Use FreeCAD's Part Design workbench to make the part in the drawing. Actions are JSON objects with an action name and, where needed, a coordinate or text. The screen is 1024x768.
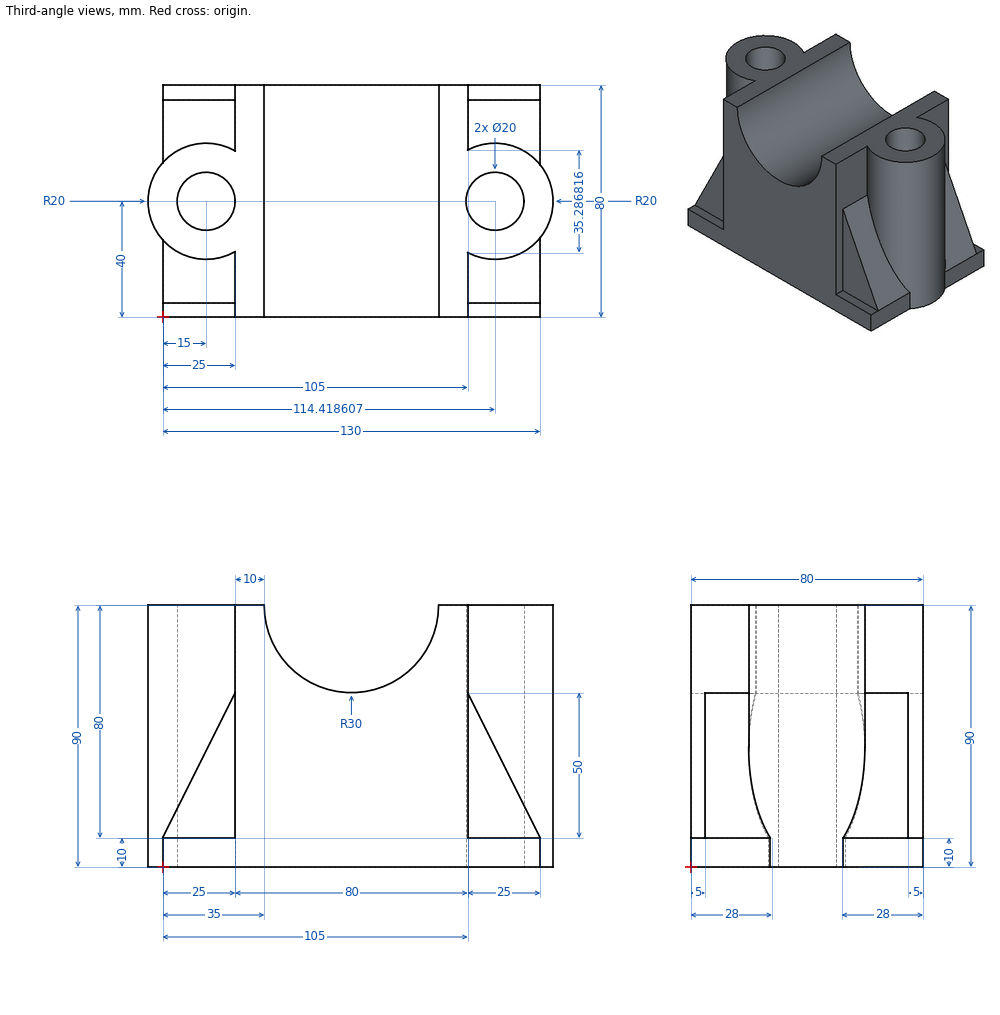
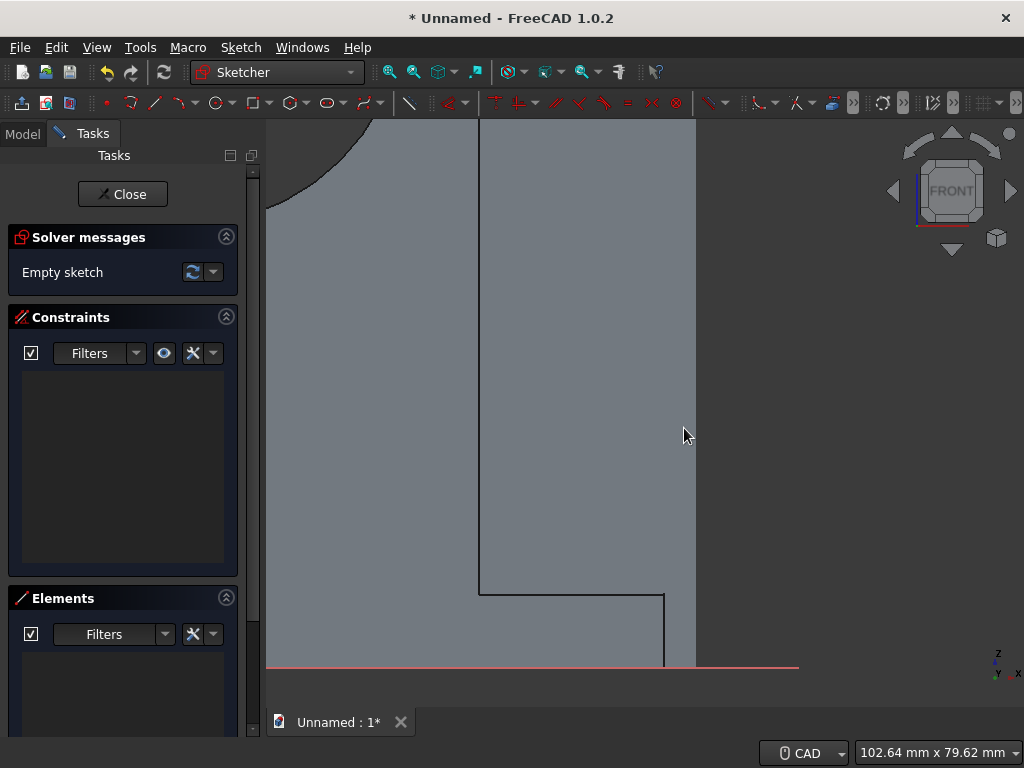
{"action": "left_click", "coordinate": [132, 104]}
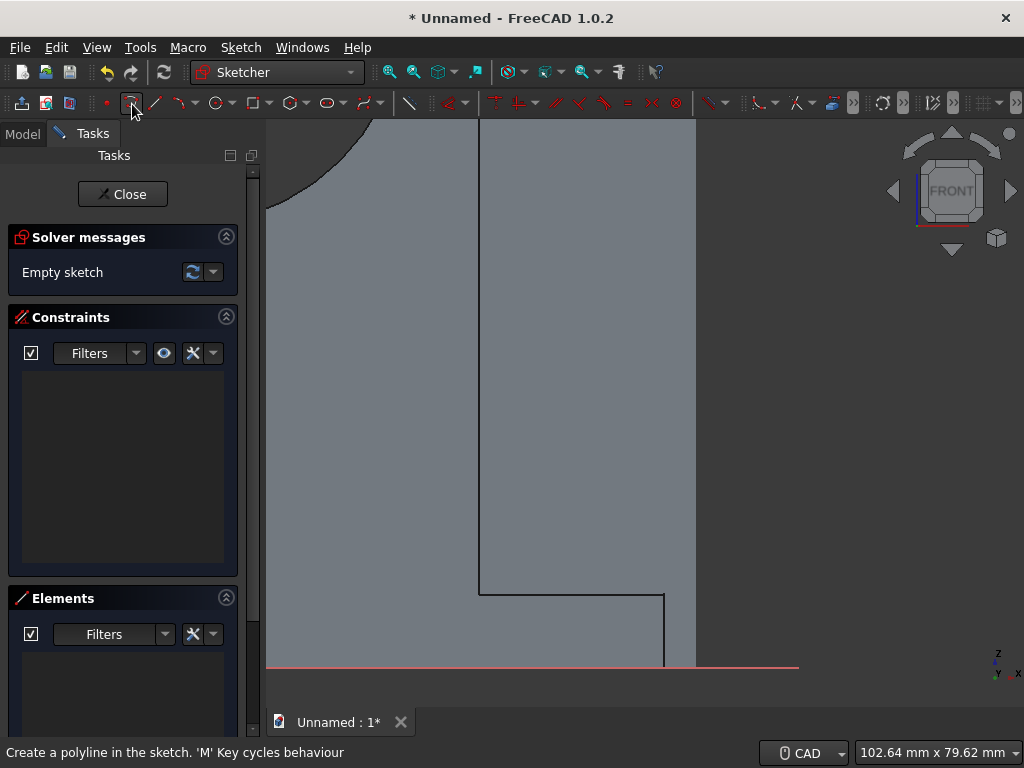
{"action": "left_click", "coordinate": [479, 594]}
{"action": "left_click", "coordinate": [664, 594]}
{"action": "left_click", "coordinate": [479, 225]}
{"action": "left_click", "coordinate": [479, 595]}
{"action": "key", "text": "Escape"}
{"action": "key", "text": "Escape"}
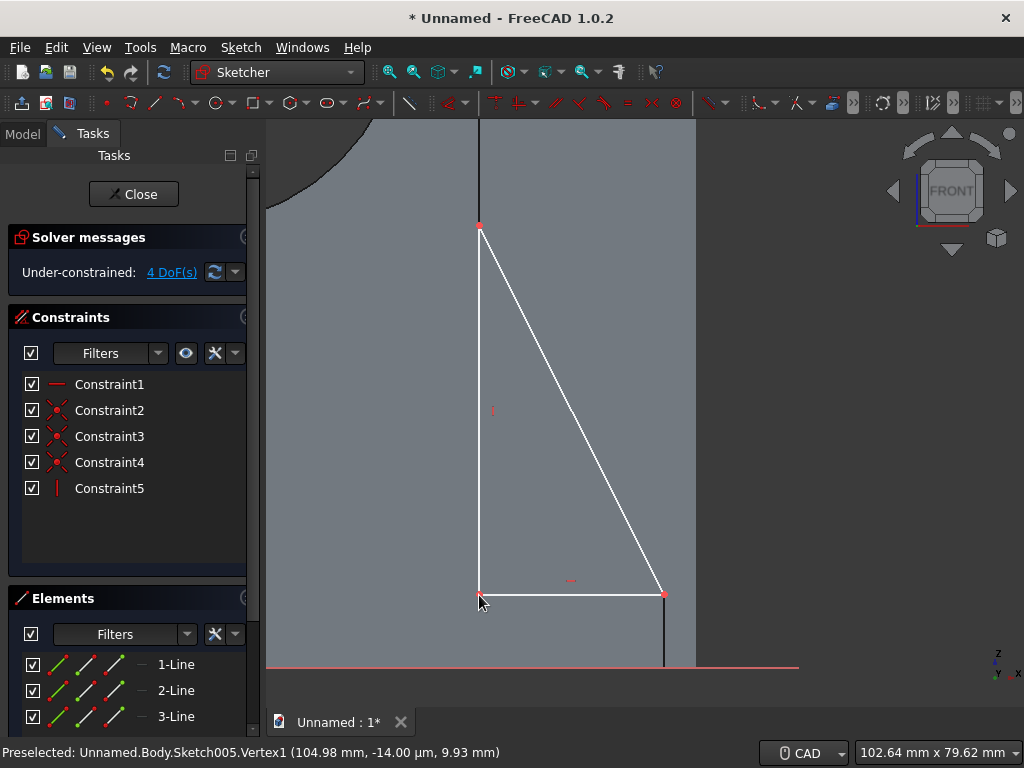
{"action": "left_click", "coordinate": [448, 104]}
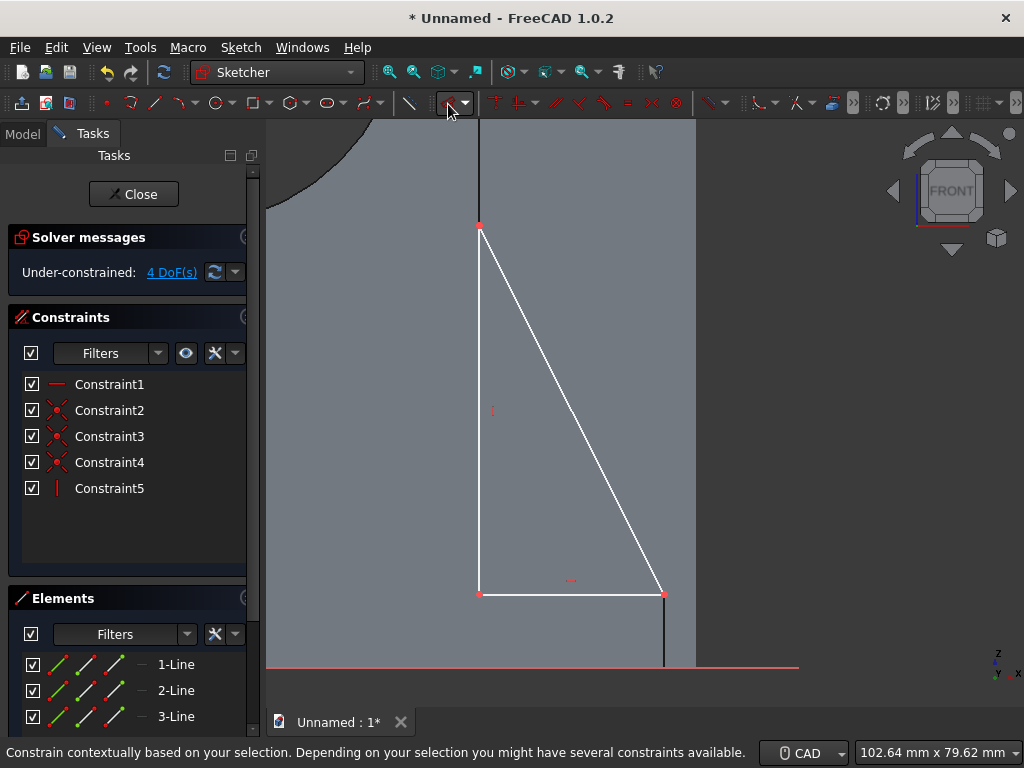
{"action": "left_click", "coordinate": [535, 595]}
{"action": "left_click", "coordinate": [572, 629]}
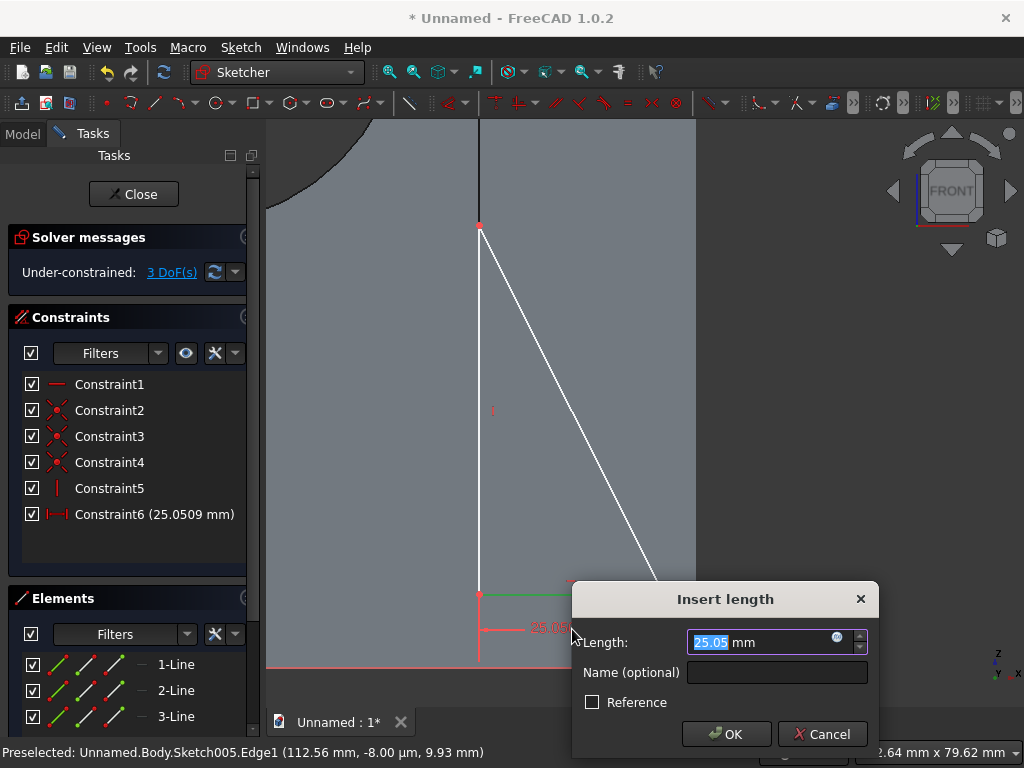
{"action": "type", "text": "25"}
{"action": "key", "text": "Return"}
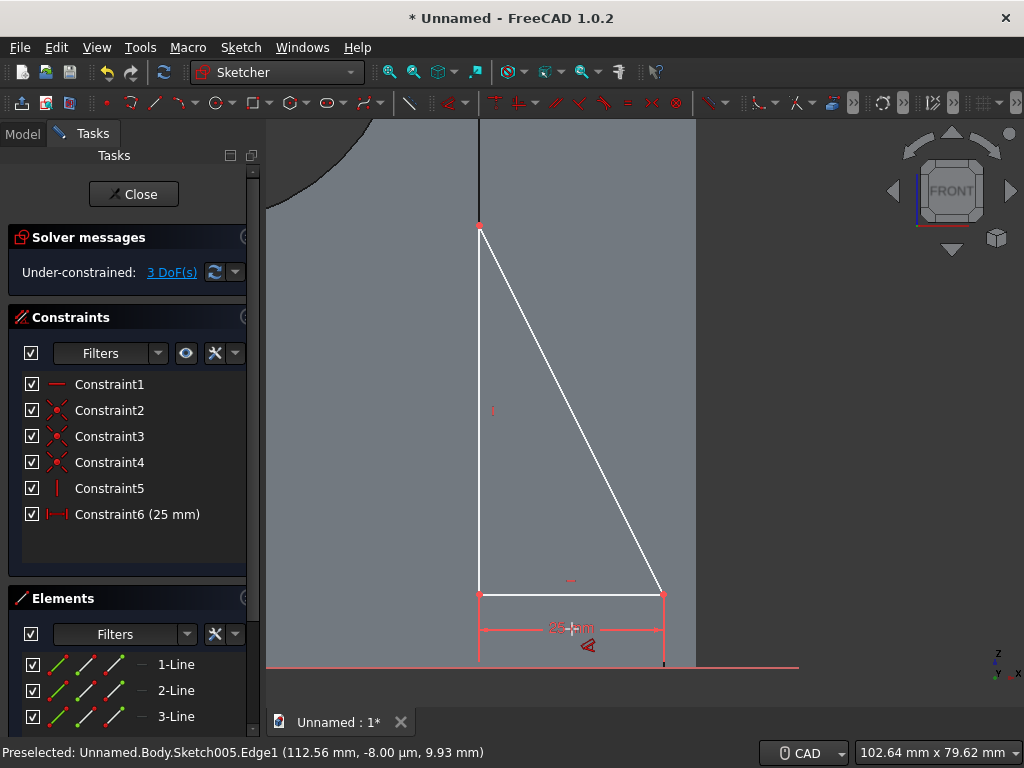
{"action": "left_click", "coordinate": [479, 337]}
{"action": "left_click", "coordinate": [445, 411]}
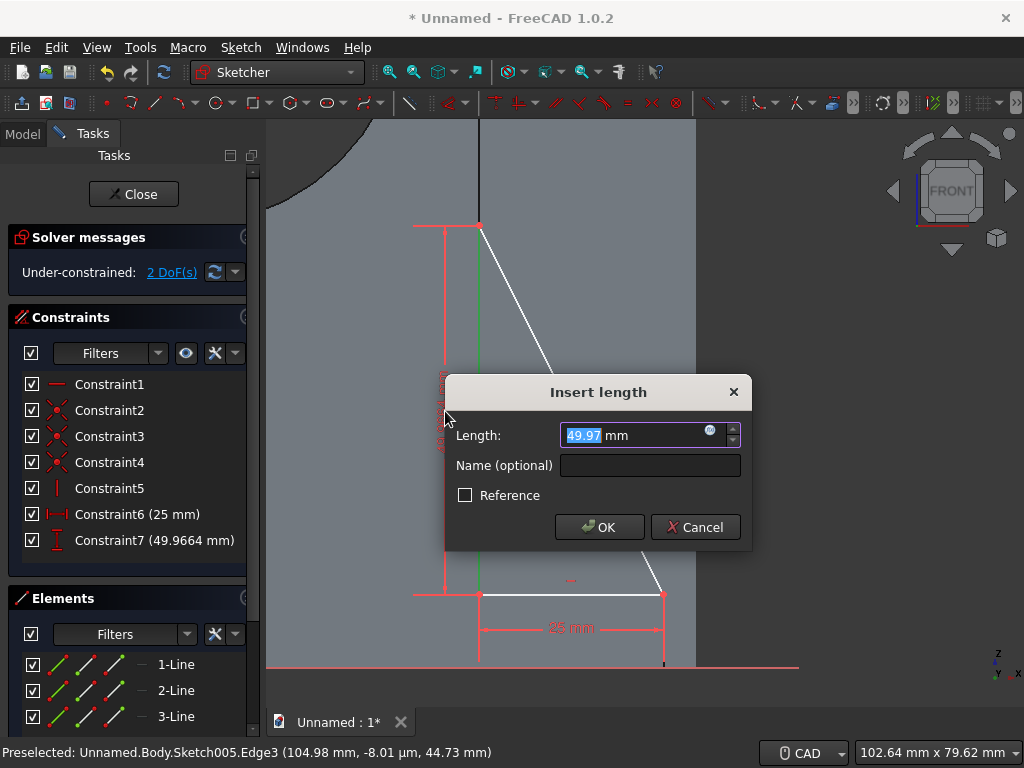
{"action": "type", "text": "50"}
{"action": "key", "text": "Return"}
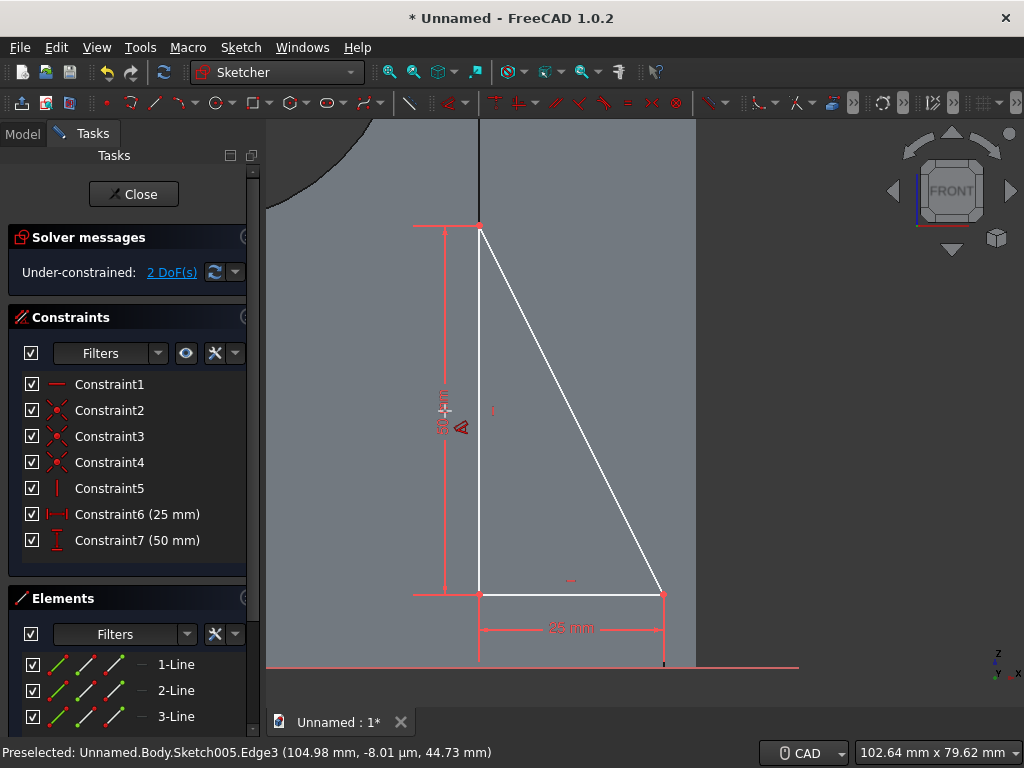
{"action": "left_click", "coordinate": [479, 595]}
{"action": "left_click", "coordinate": [659, 632]}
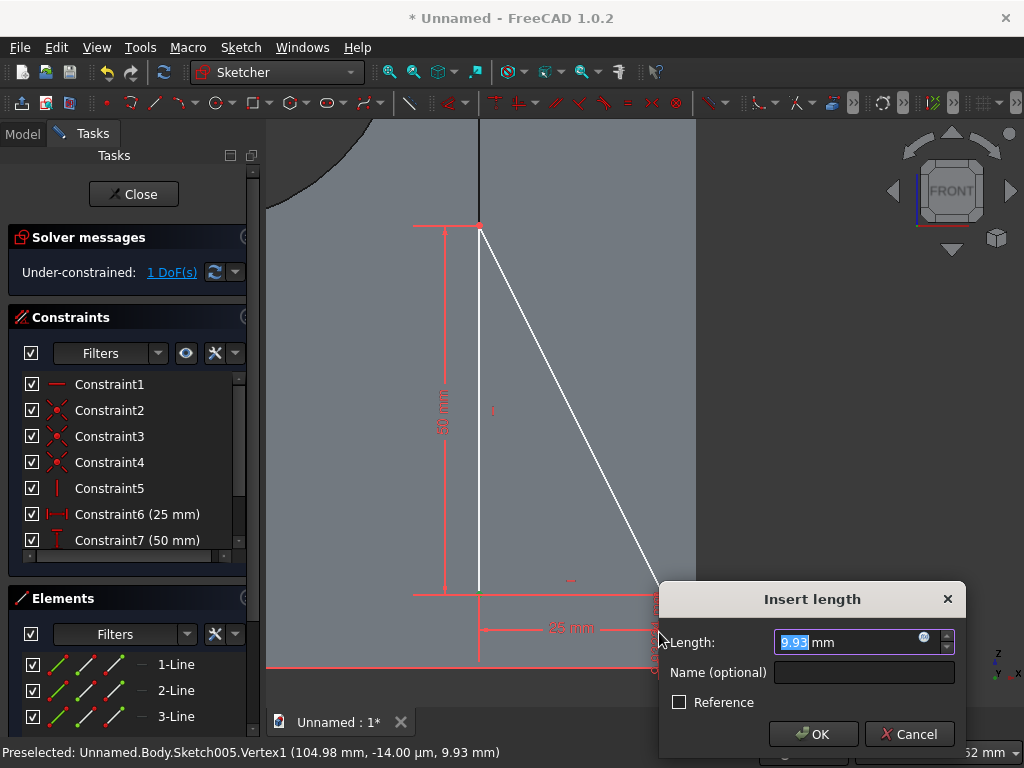
{"action": "type", "text": "10"}
{"action": "key", "text": "Return"}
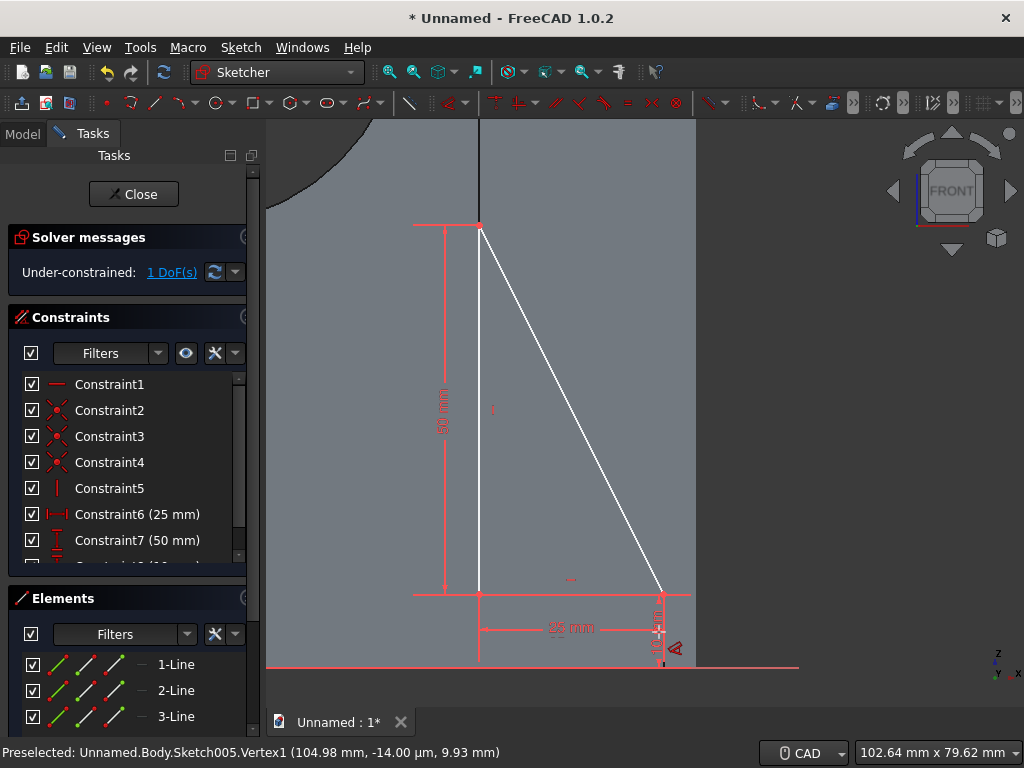
{"action": "left_click", "coordinate": [479, 594]}
{"action": "left_click", "coordinate": [386, 560]}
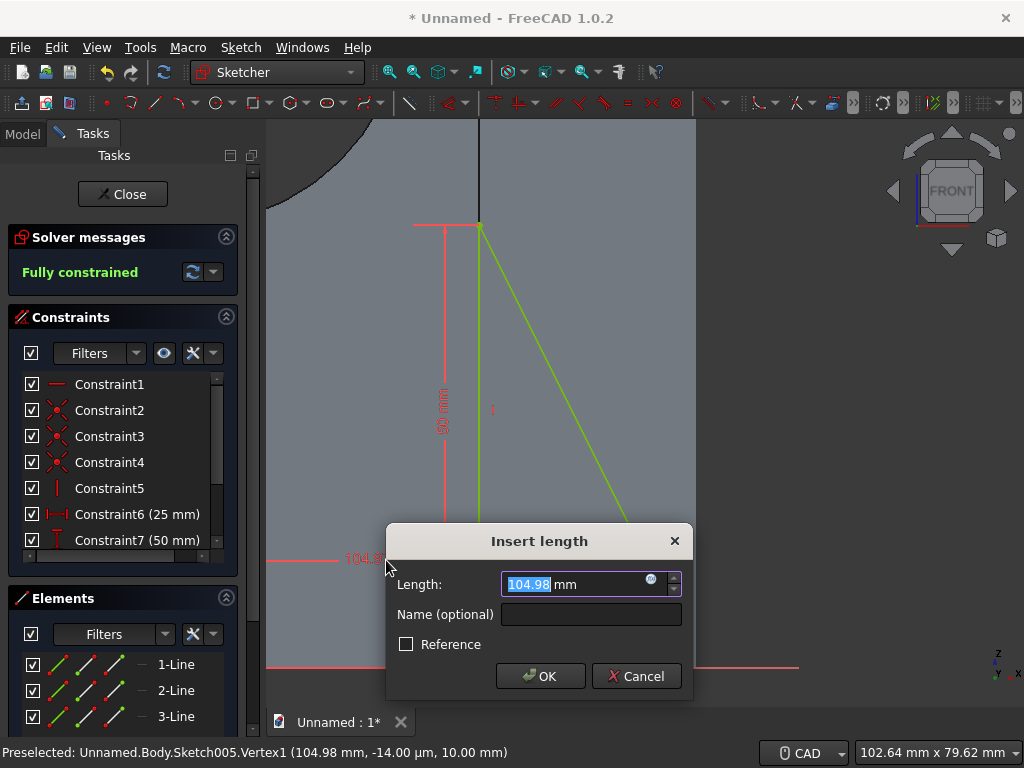
{"action": "type", "text": "105"}
{"action": "key", "text": "Return"}
{"action": "key", "text": "Escape"}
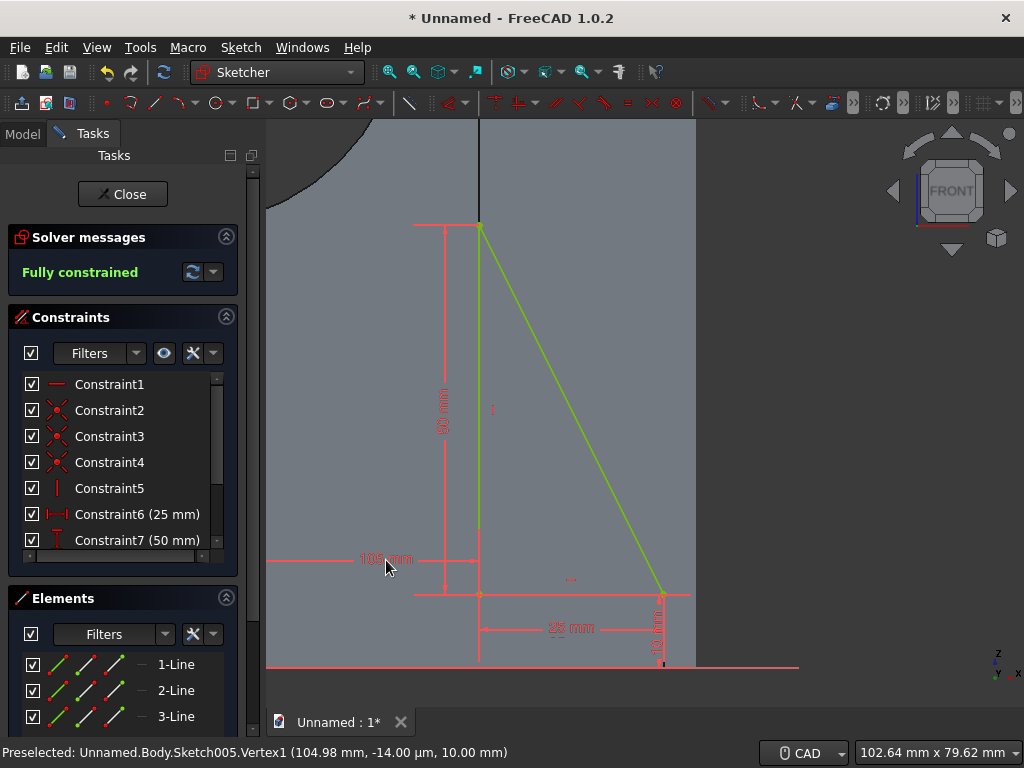
{"action": "left_click", "coordinate": [123, 194]}